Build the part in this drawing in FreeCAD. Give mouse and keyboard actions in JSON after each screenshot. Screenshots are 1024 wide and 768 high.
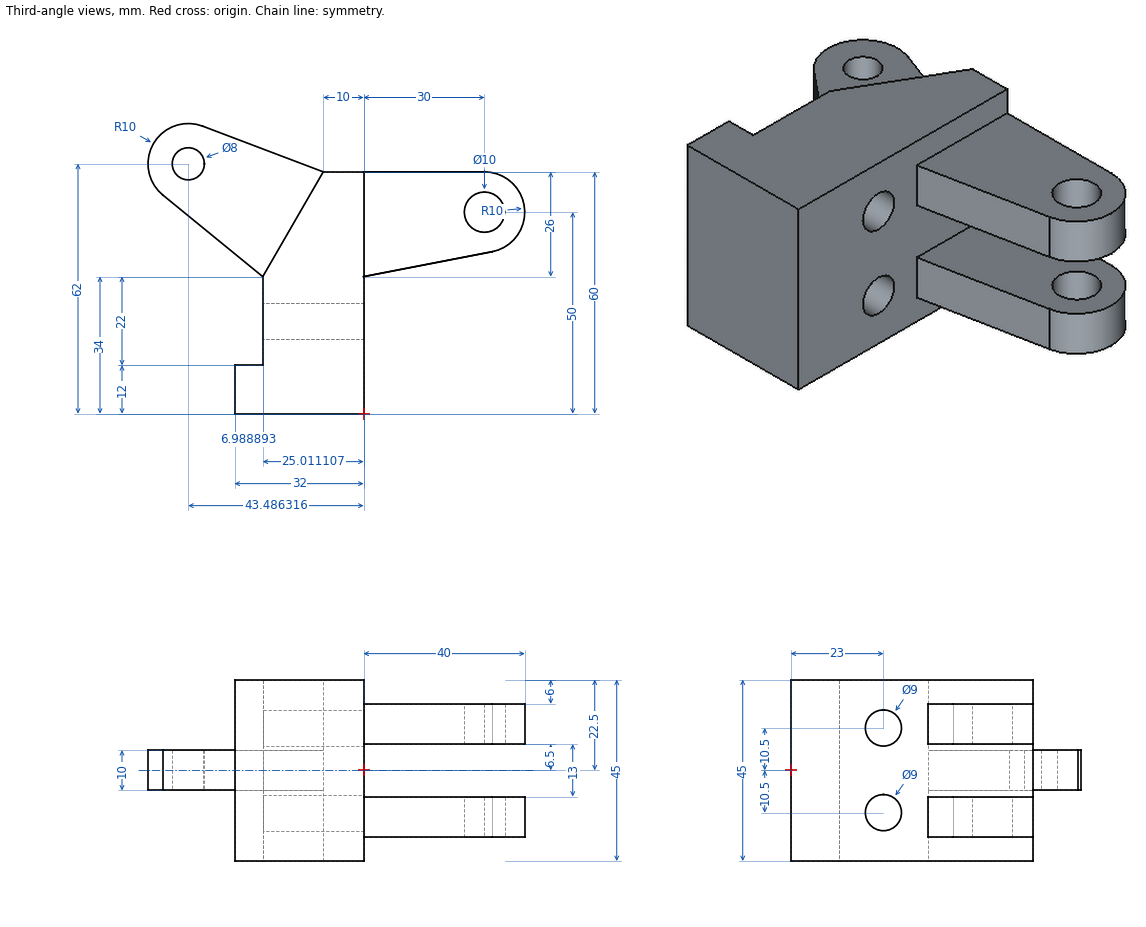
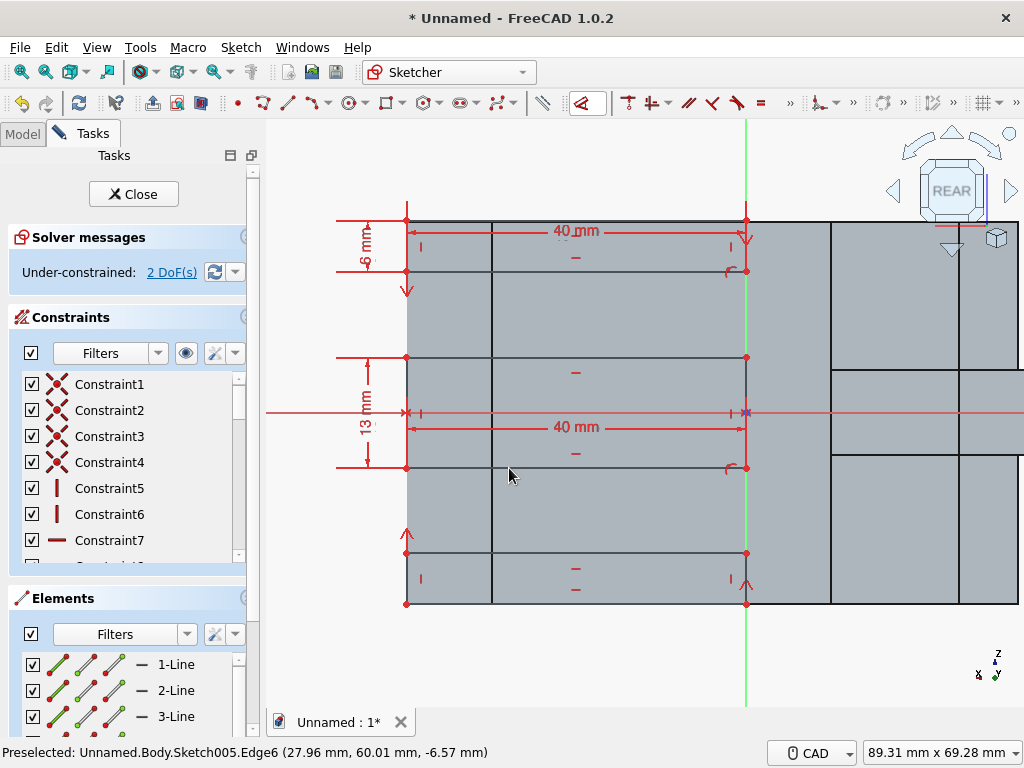
{"action": "left_click", "coordinate": [407, 358]}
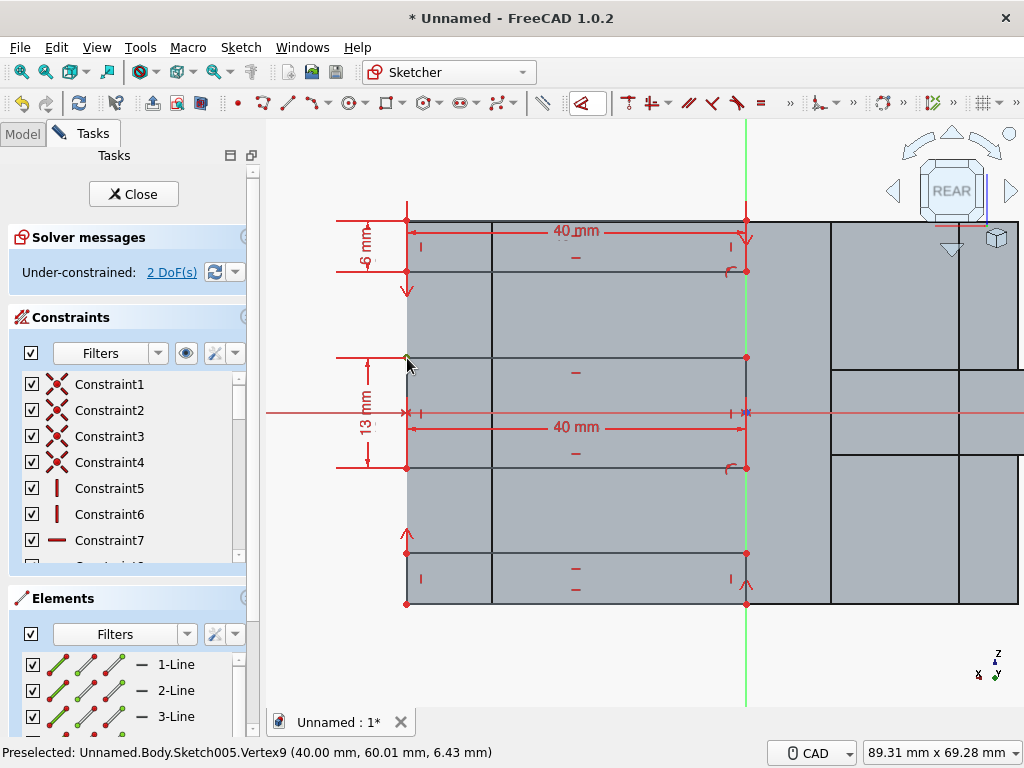
{"action": "key", "text": "i"}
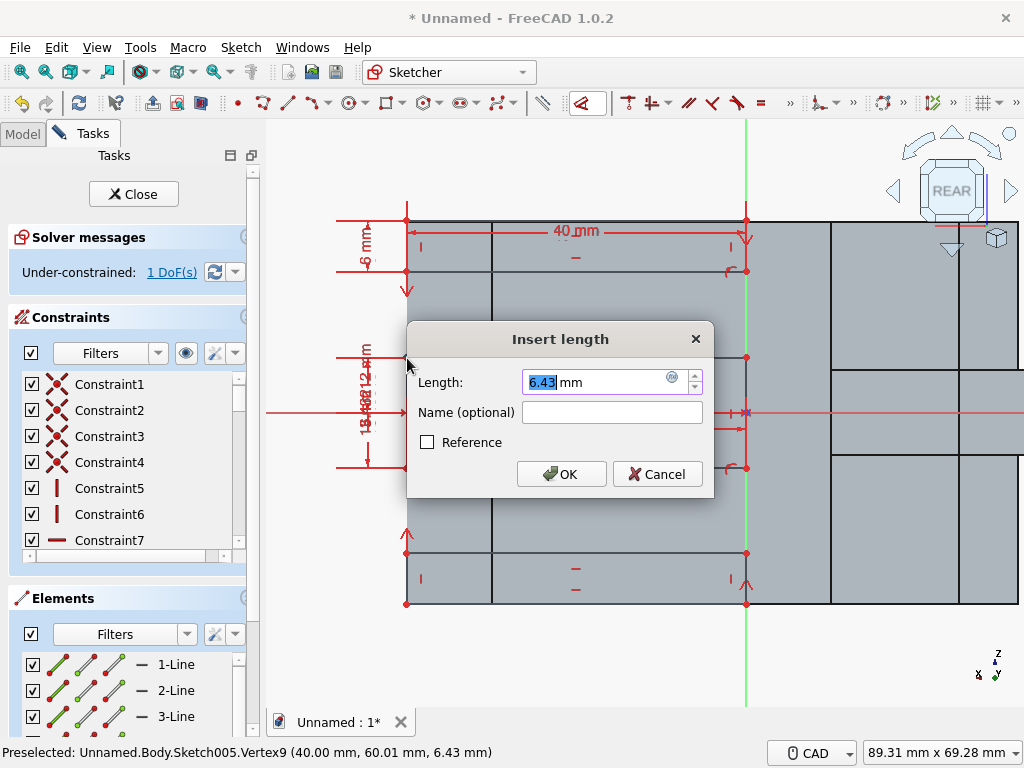
{"action": "type", "text": "6.5"}
{"action": "key", "text": "Return"}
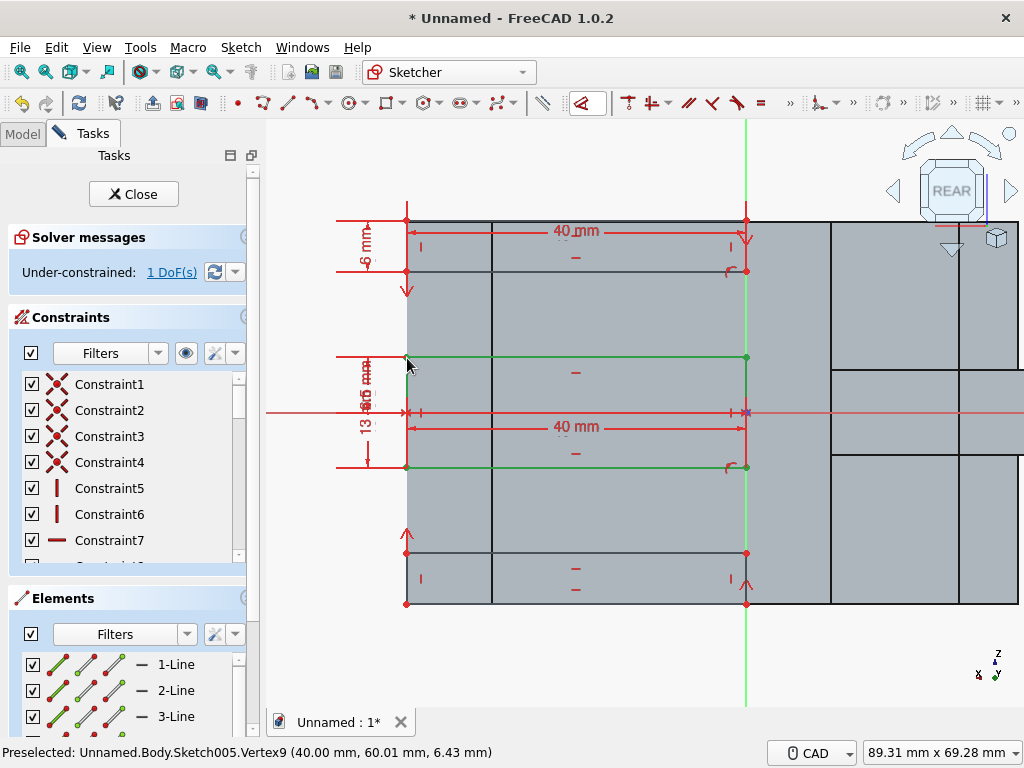
{"action": "left_click", "coordinate": [407, 221]}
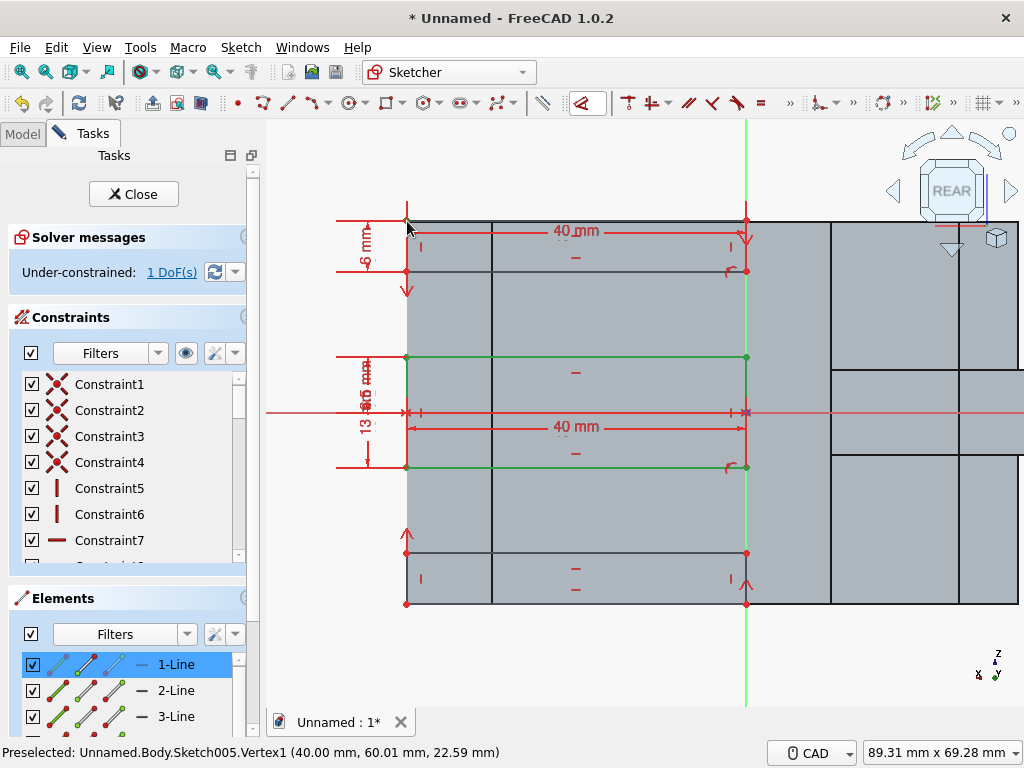
{"action": "key", "text": "i"}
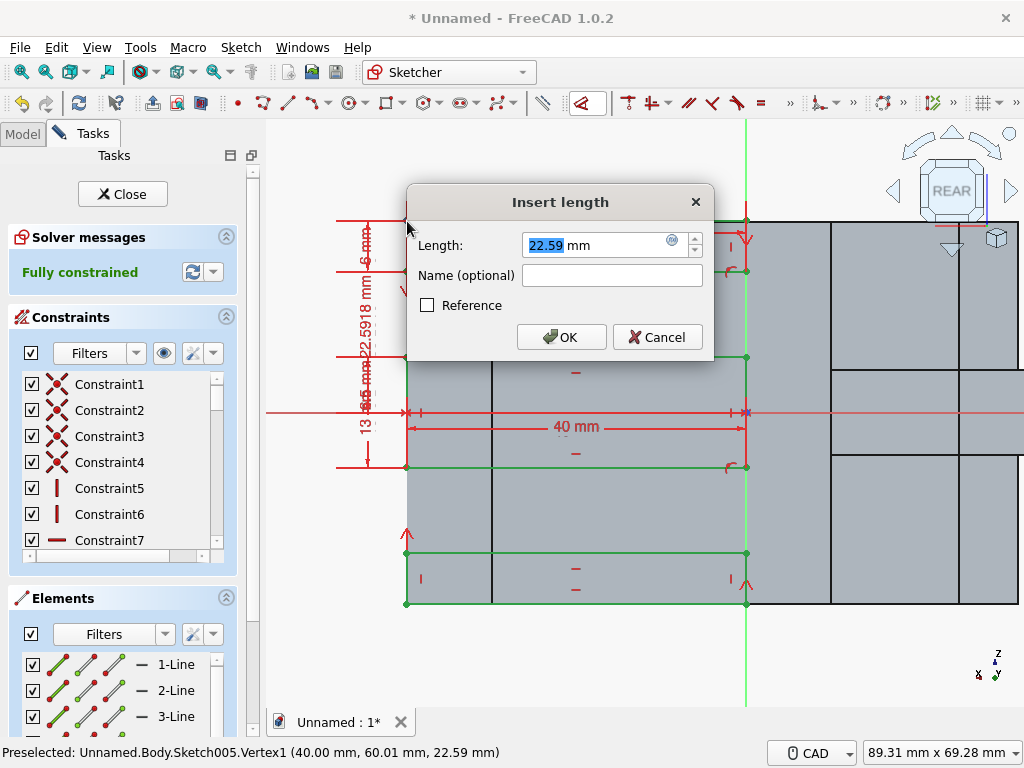
{"action": "type", "text": "22.5"}
{"action": "key", "text": "Return"}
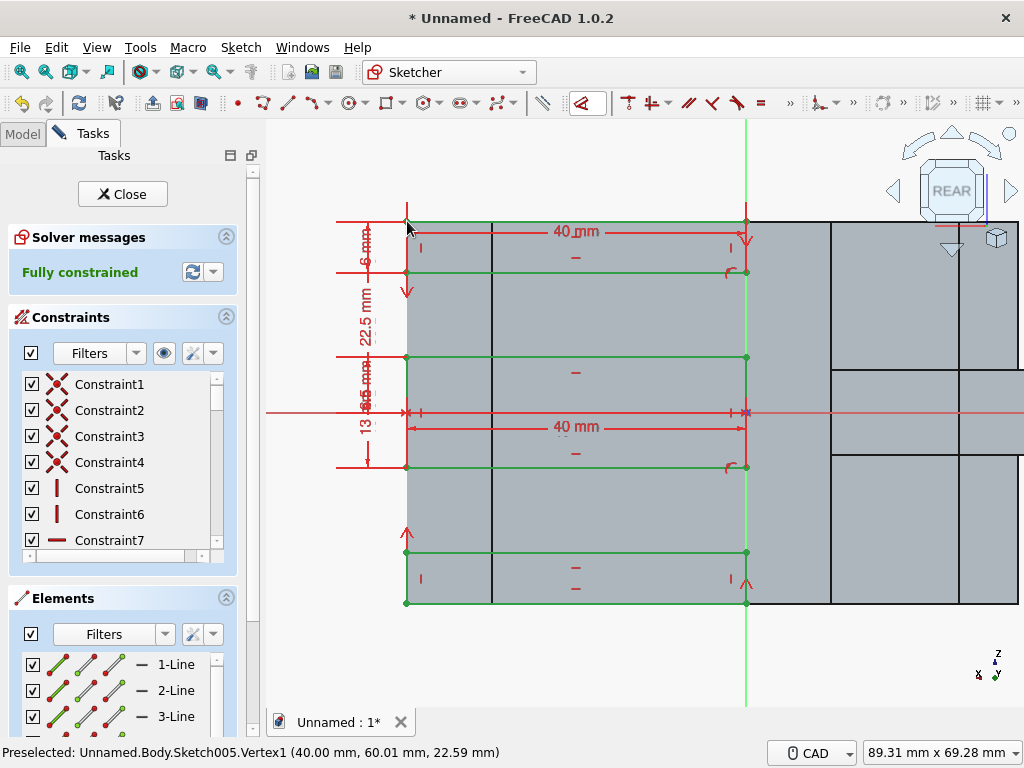
{"action": "left_click", "coordinate": [123, 194]}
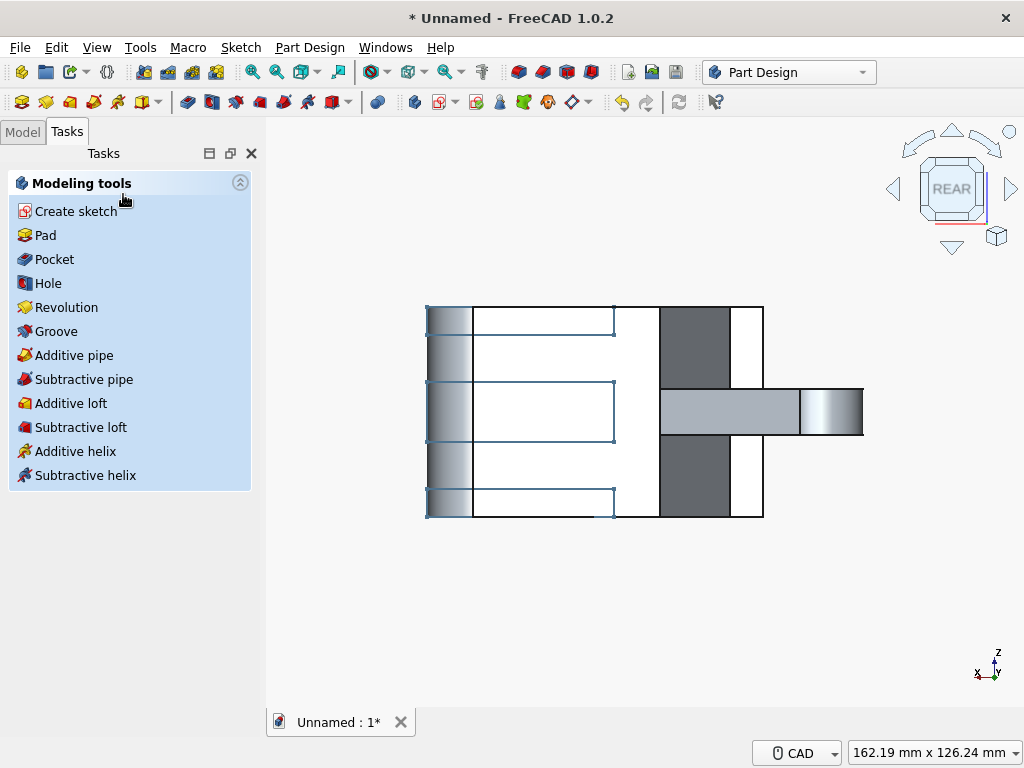
{"action": "left_click", "coordinate": [188, 102]}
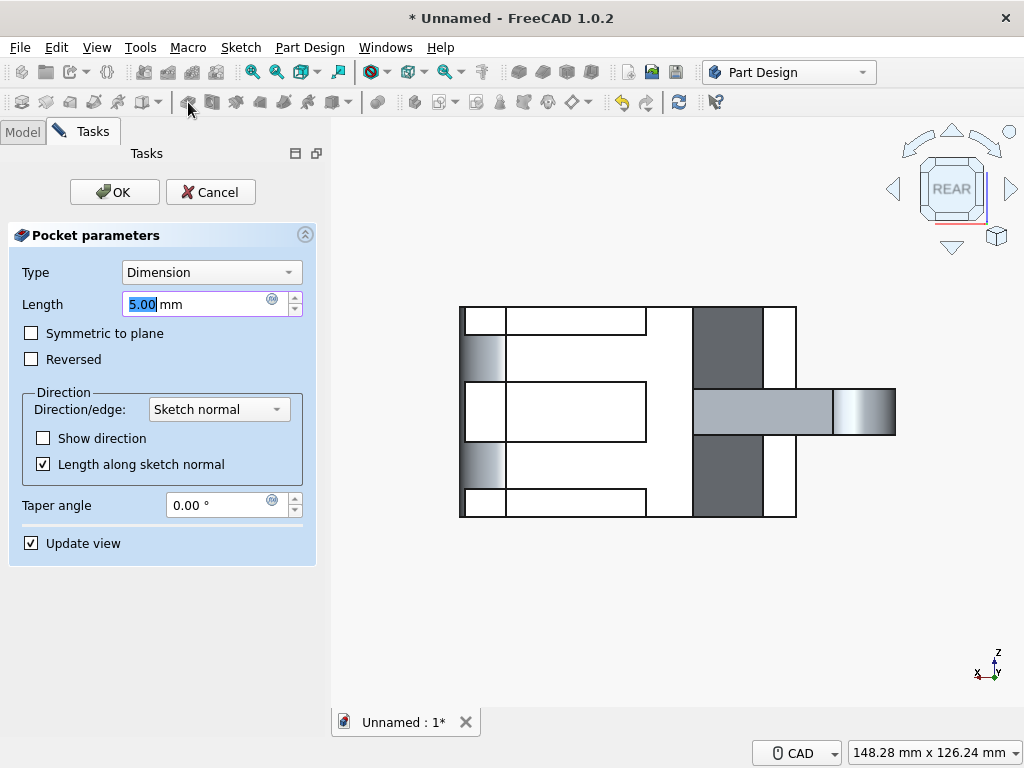
{"action": "left_click", "coordinate": [212, 272]}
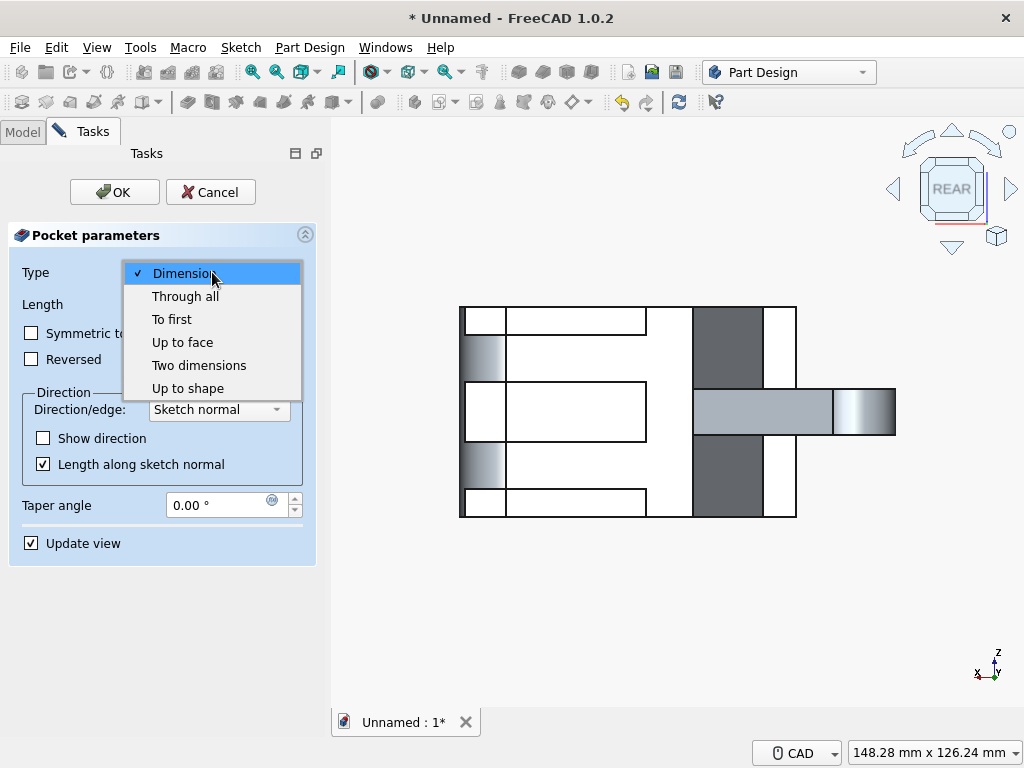
{"action": "left_click", "coordinate": [212, 296]}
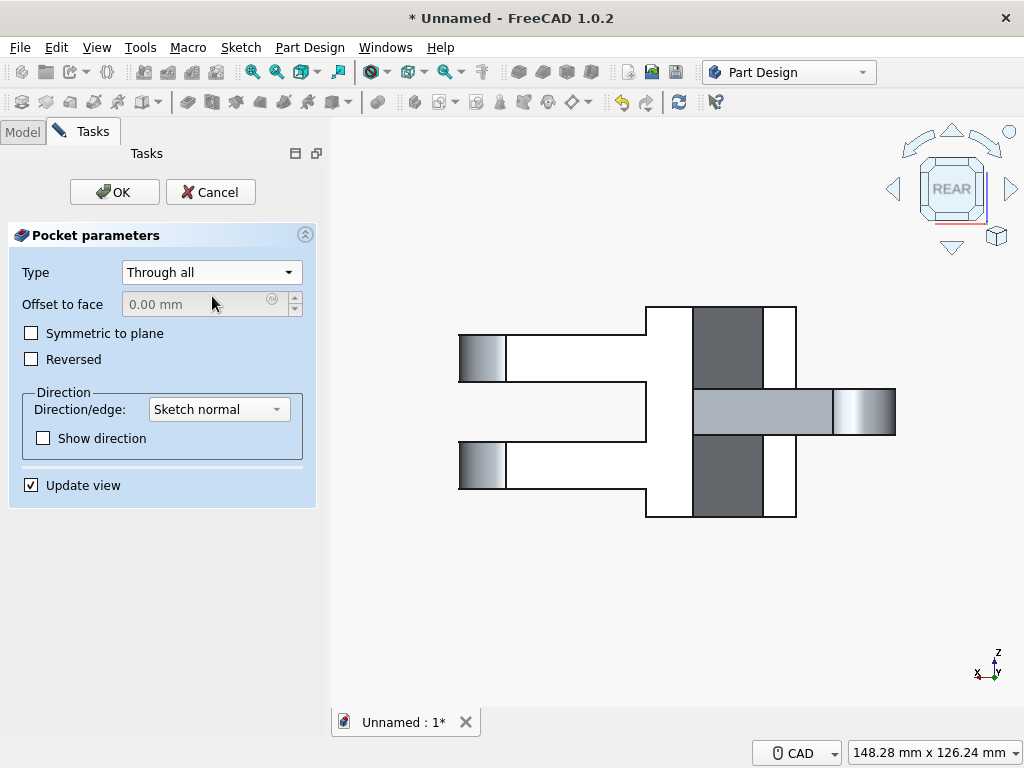
{"action": "left_click", "coordinate": [115, 192]}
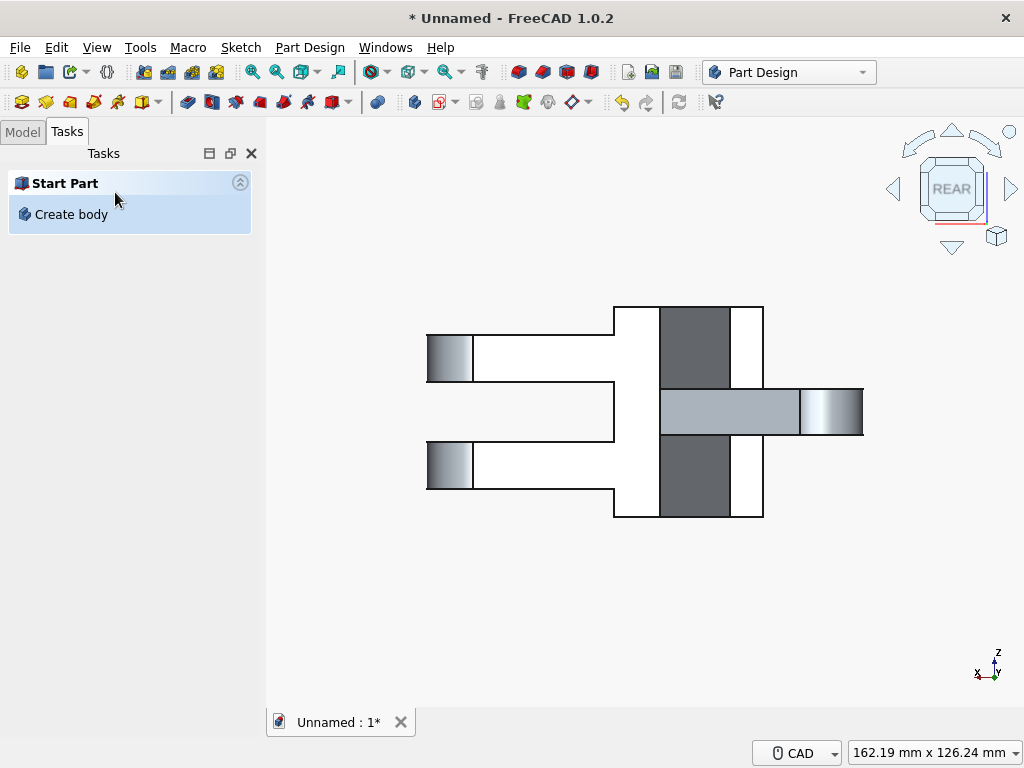
{"action": "key", "text": "0"}